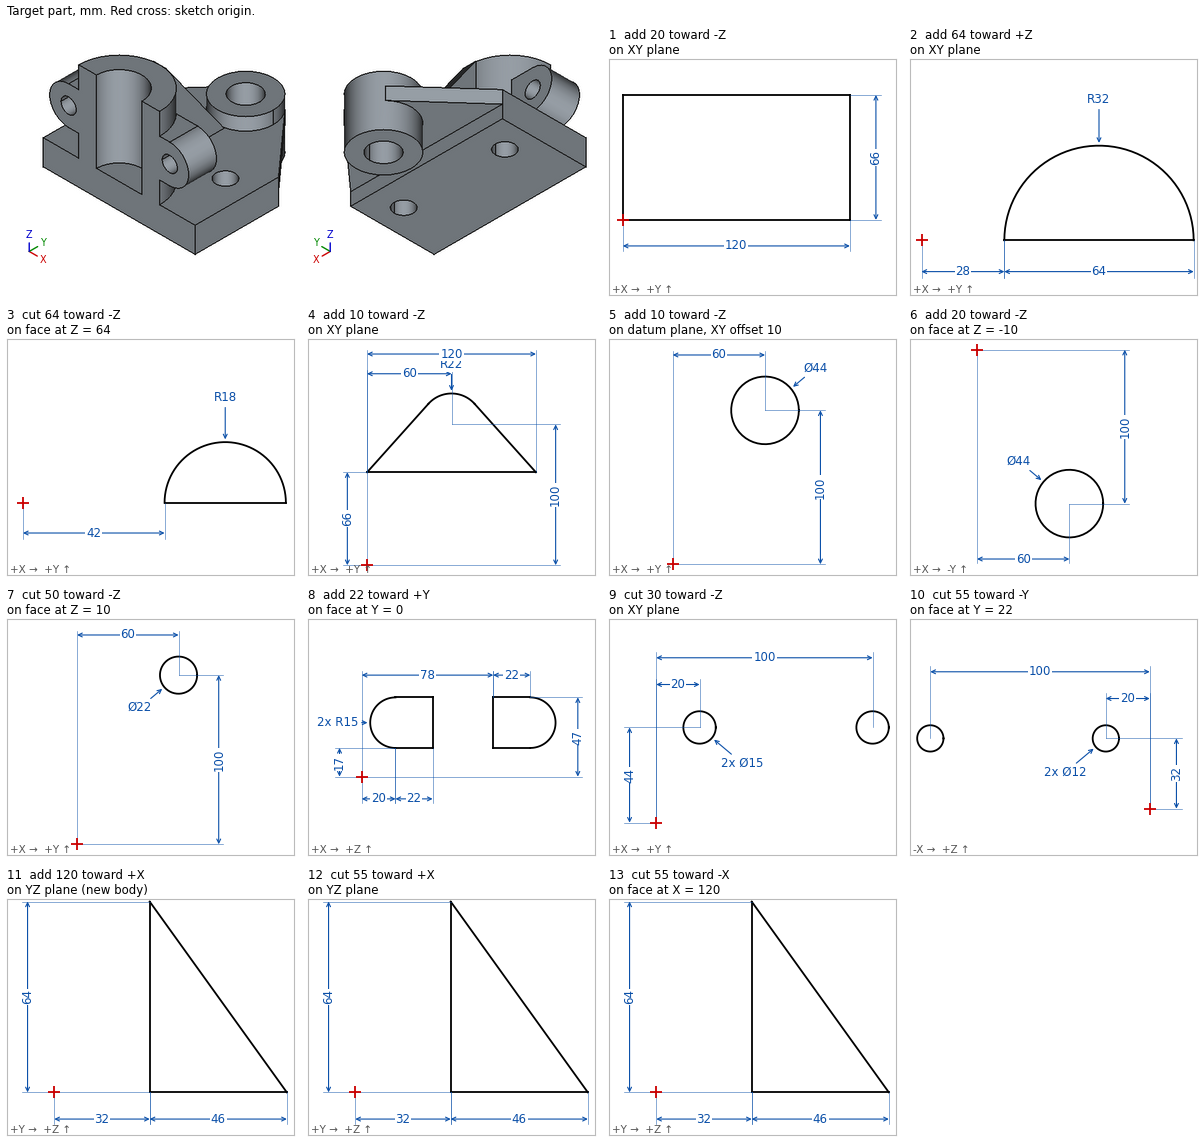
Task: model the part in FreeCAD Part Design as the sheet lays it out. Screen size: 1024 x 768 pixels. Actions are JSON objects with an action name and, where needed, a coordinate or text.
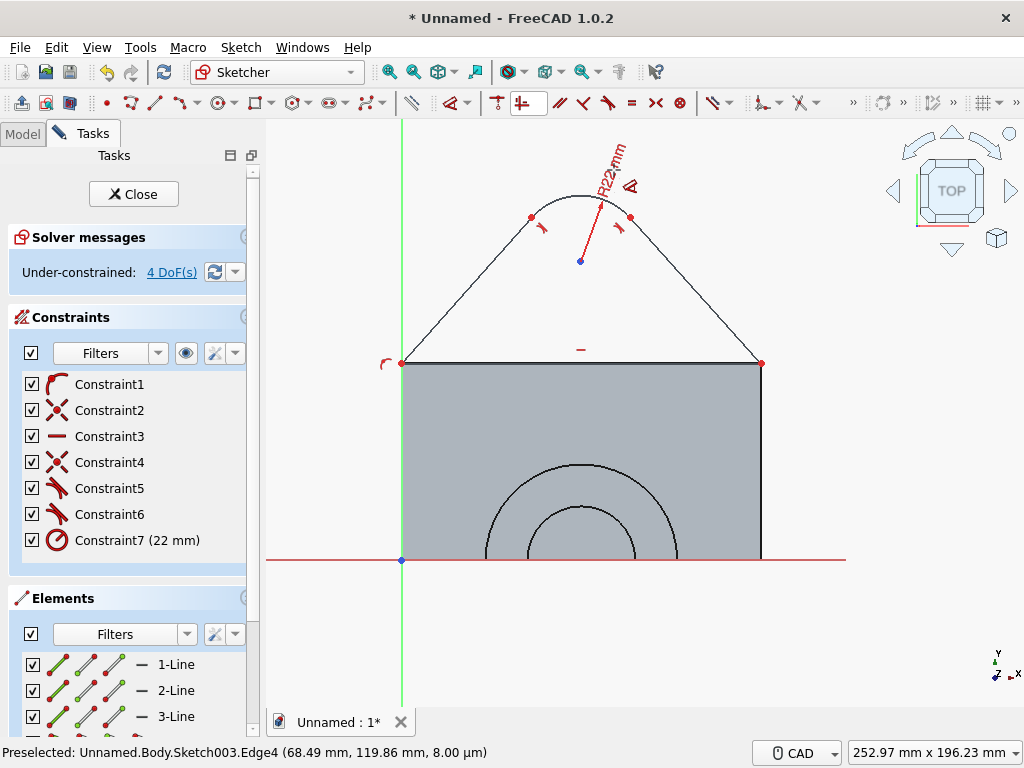
{"action": "left_click", "coordinate": [509, 364]}
{"action": "left_click", "coordinate": [581, 330]}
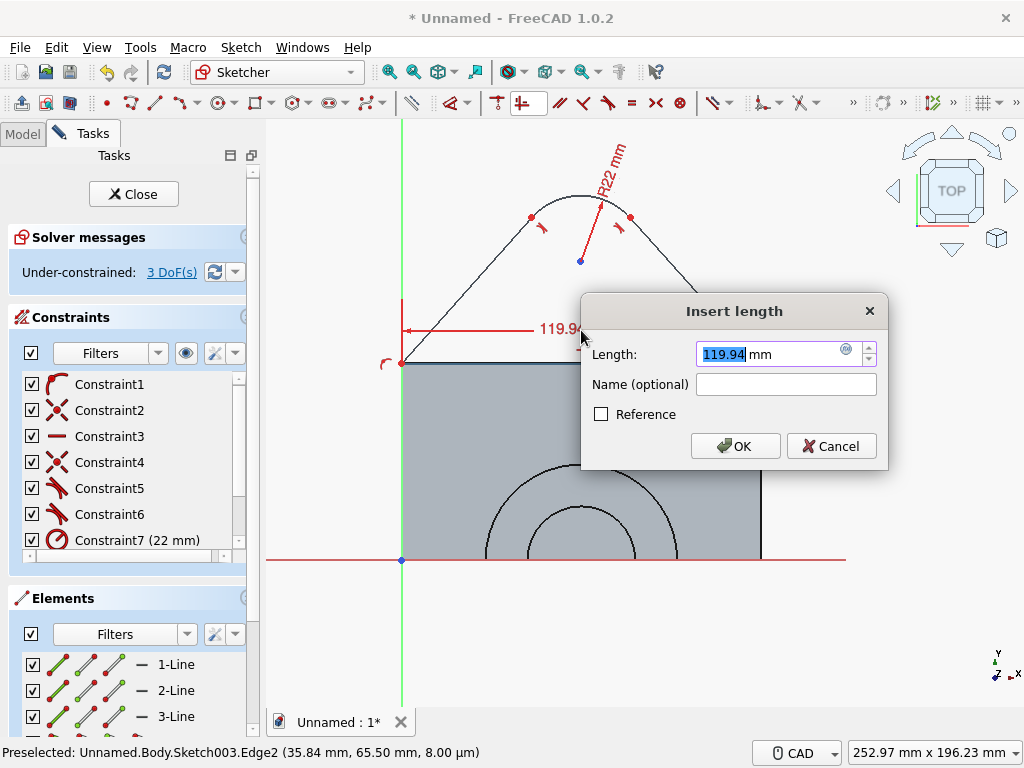
{"action": "type", "text": "120"}
{"action": "key", "text": "Return"}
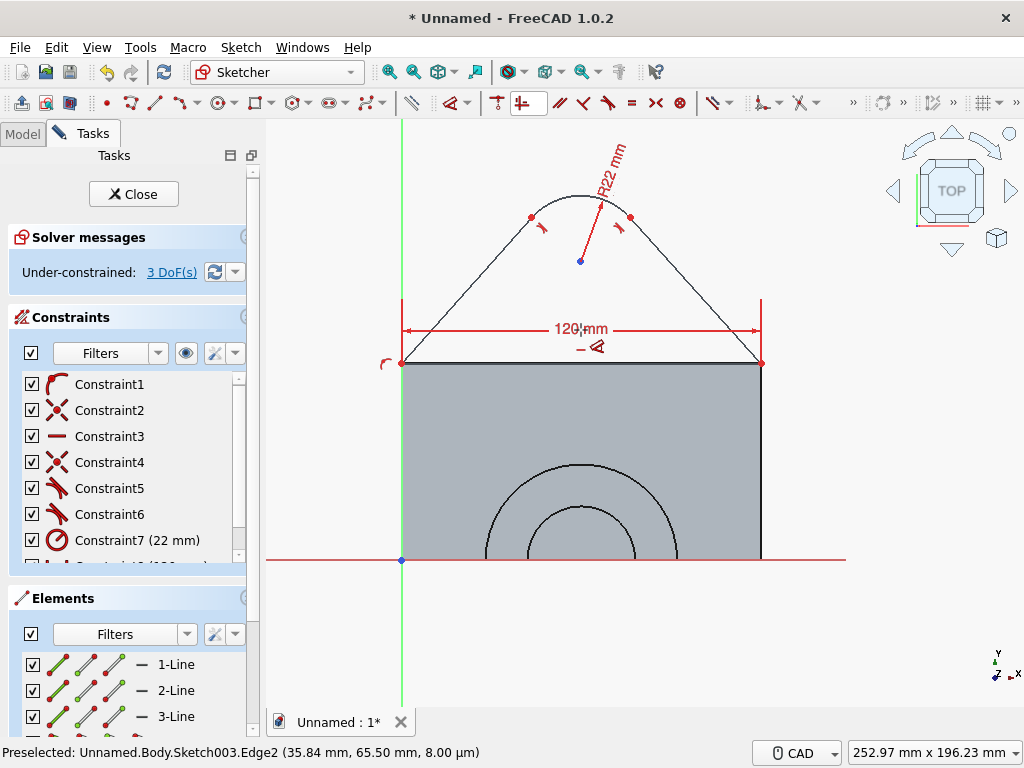
{"action": "left_click", "coordinate": [402, 364]}
{"action": "left_click", "coordinate": [368, 462]}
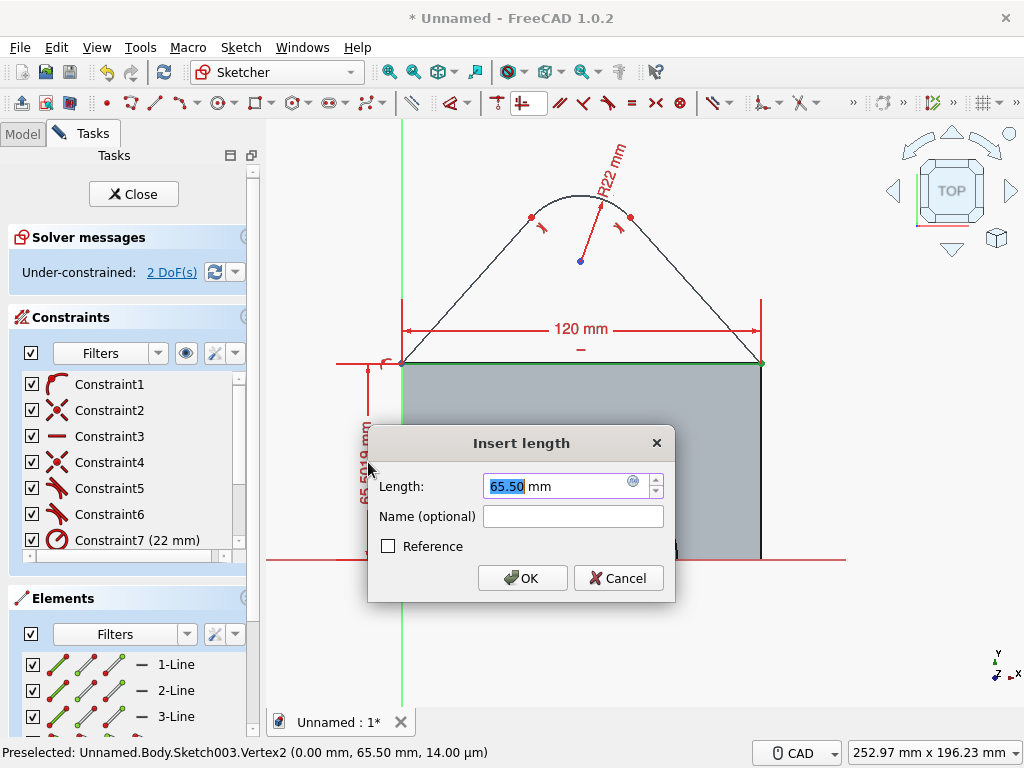
{"action": "type", "text": "66"}
{"action": "key", "text": "Return"}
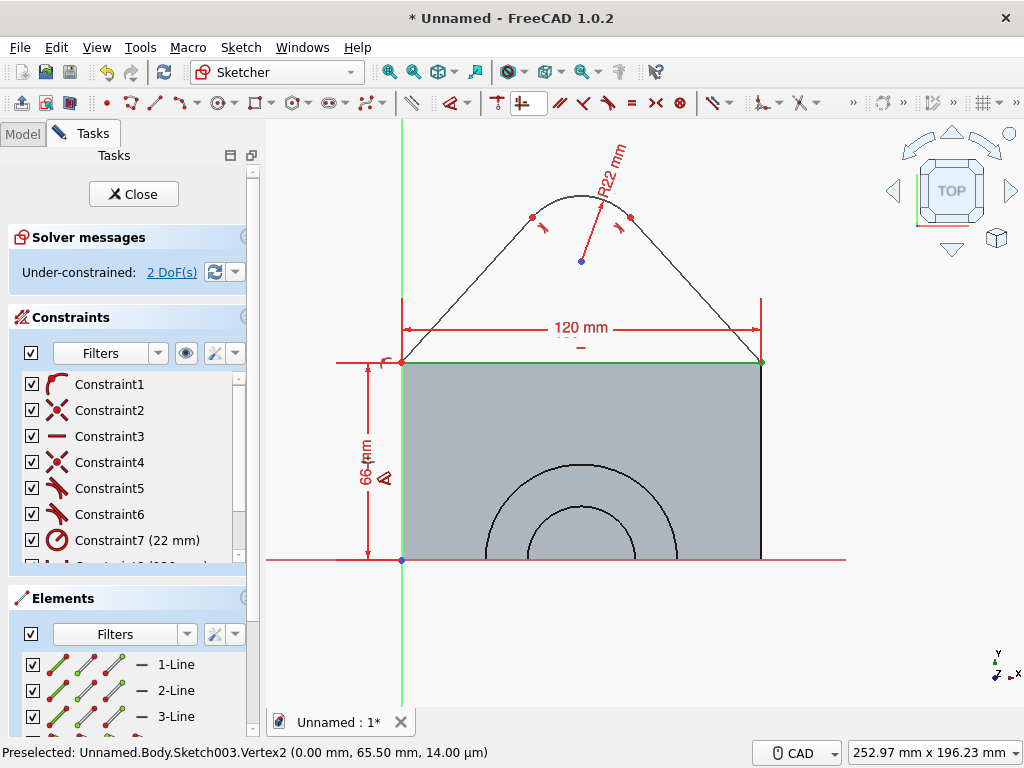
{"action": "left_click", "coordinate": [581, 262]}
{"action": "left_click", "coordinate": [491, 594]}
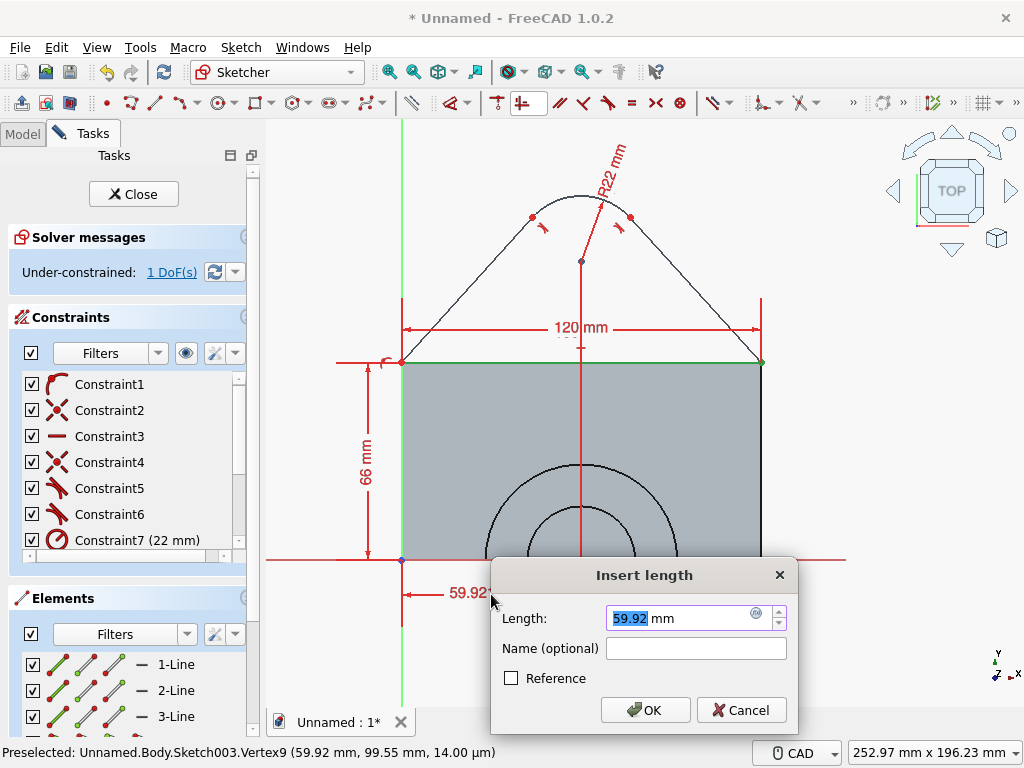
{"action": "type", "text": "60"}
{"action": "key", "text": "Return"}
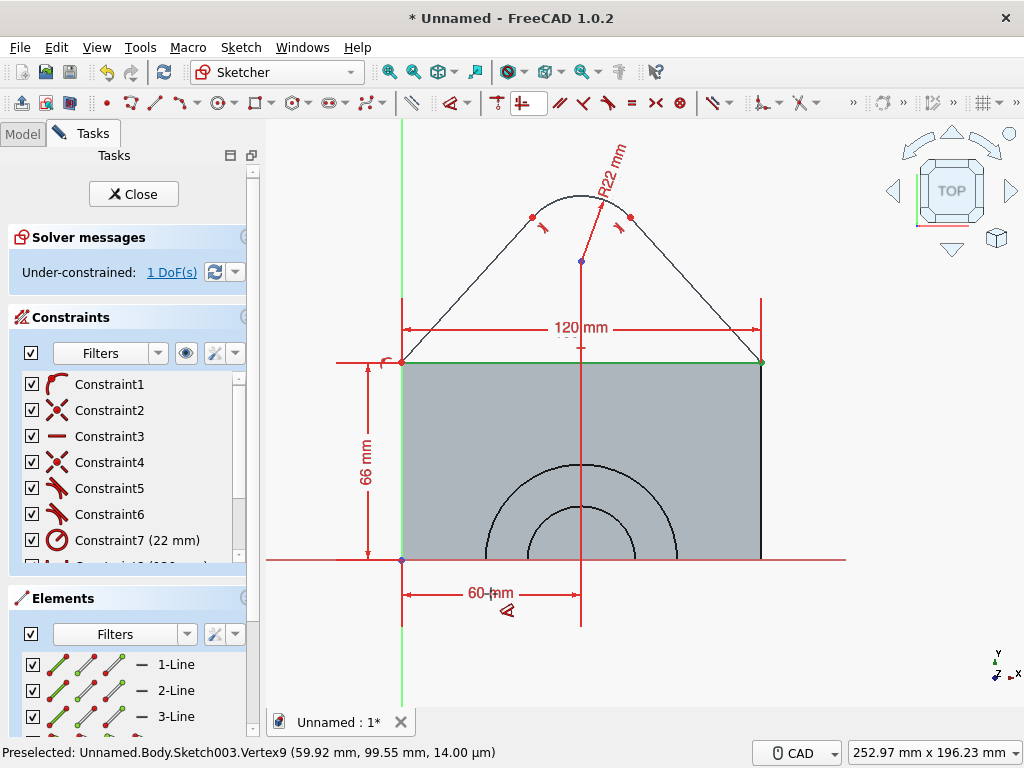
{"action": "left_click", "coordinate": [581, 262]}
{"action": "left_click", "coordinate": [368, 411]}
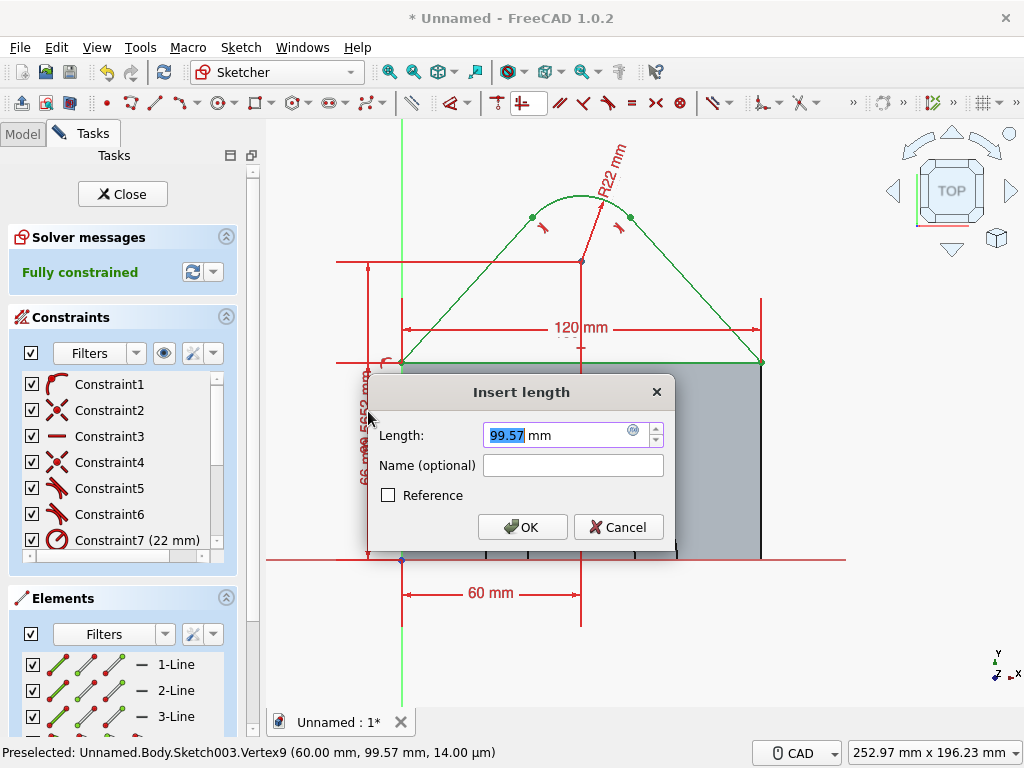
{"action": "type", "text": "100"}
{"action": "key", "text": "Return"}
{"action": "key", "text": "Escape"}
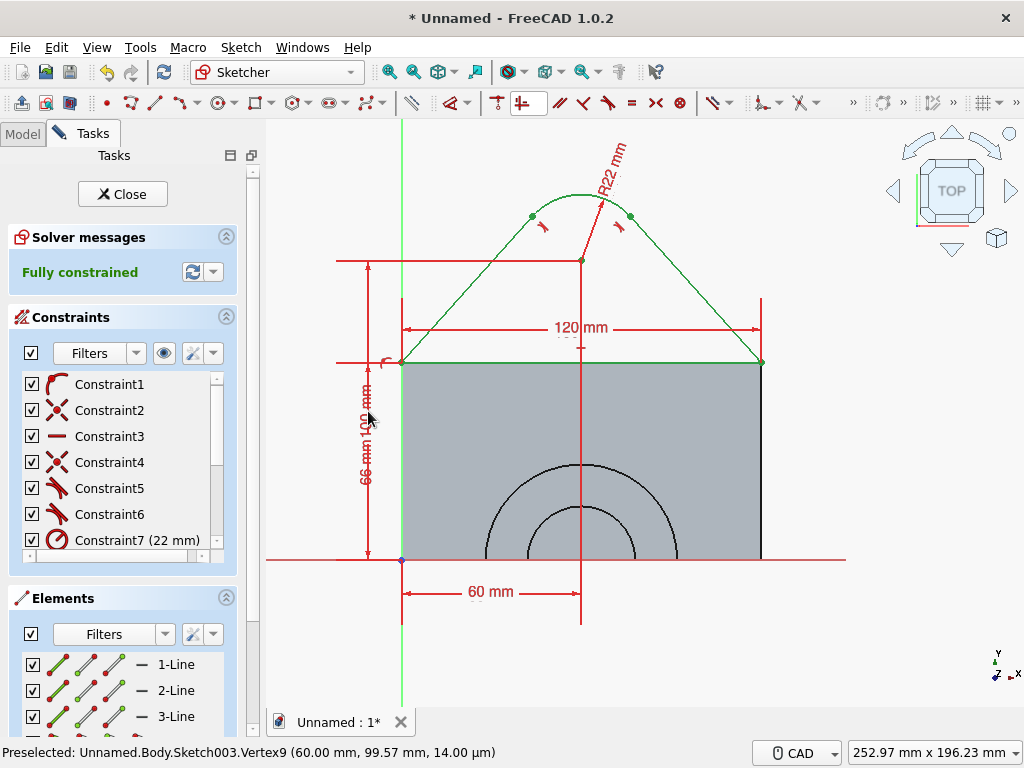
{"action": "left_click", "coordinate": [123, 194]}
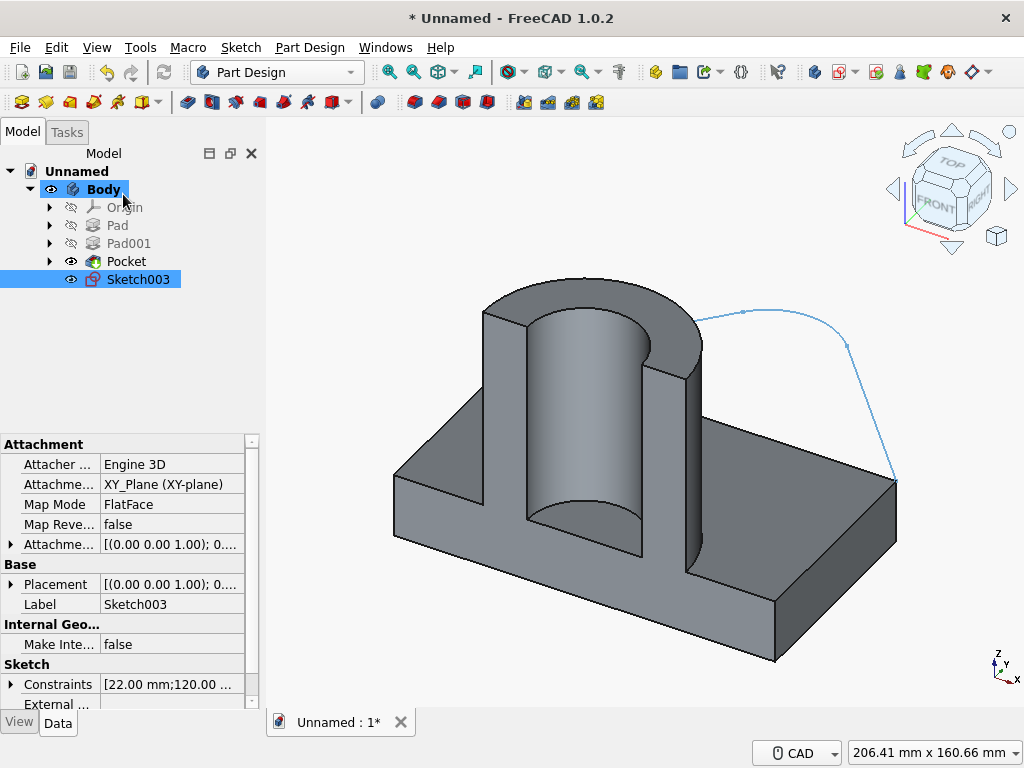
{"action": "left_click", "coordinate": [22, 102]}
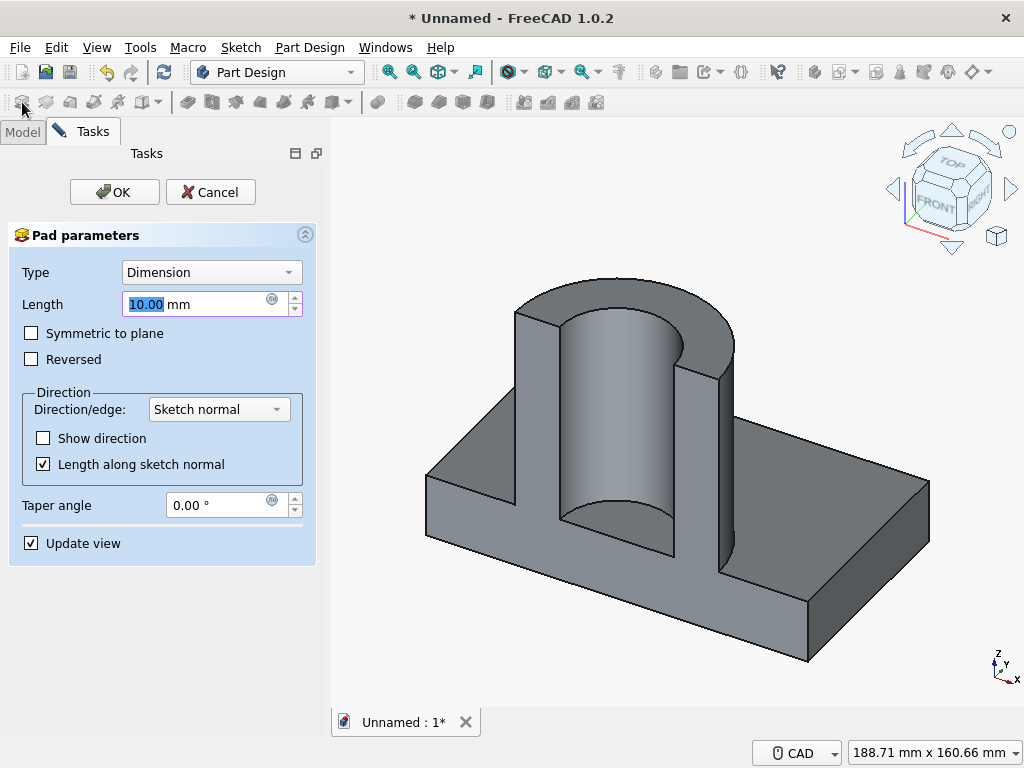
{"action": "type", "text": "10"}
{"action": "key", "text": "Tab"}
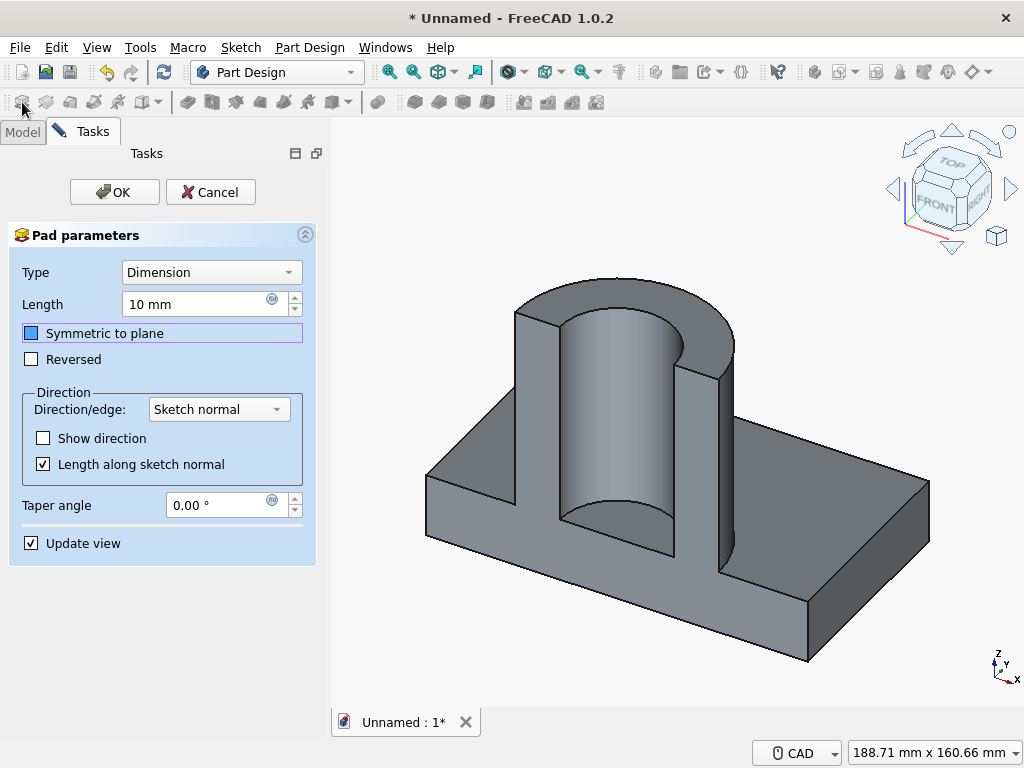
{"action": "left_click", "coordinate": [30, 359]}